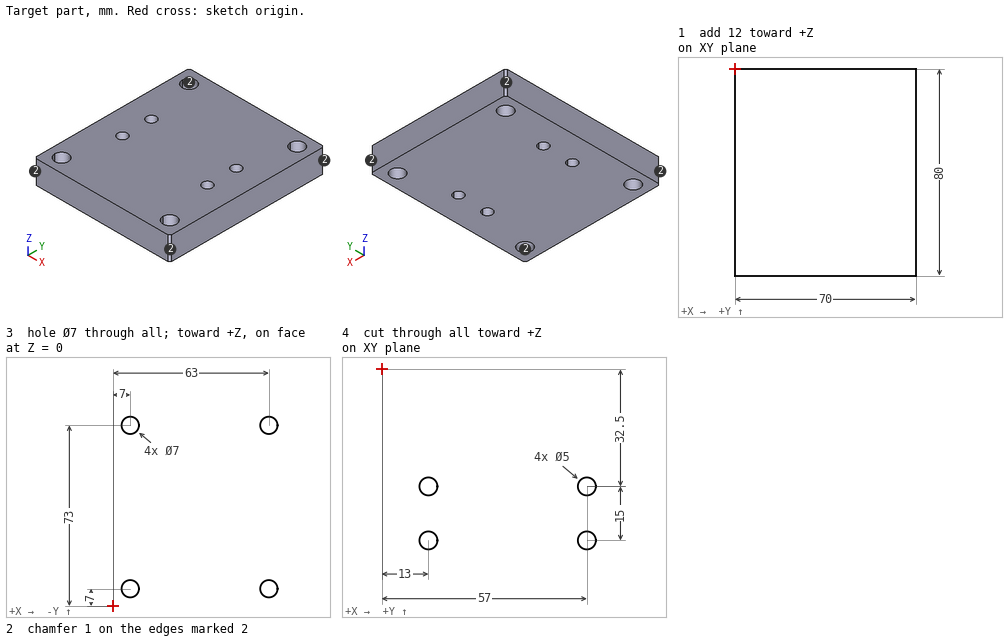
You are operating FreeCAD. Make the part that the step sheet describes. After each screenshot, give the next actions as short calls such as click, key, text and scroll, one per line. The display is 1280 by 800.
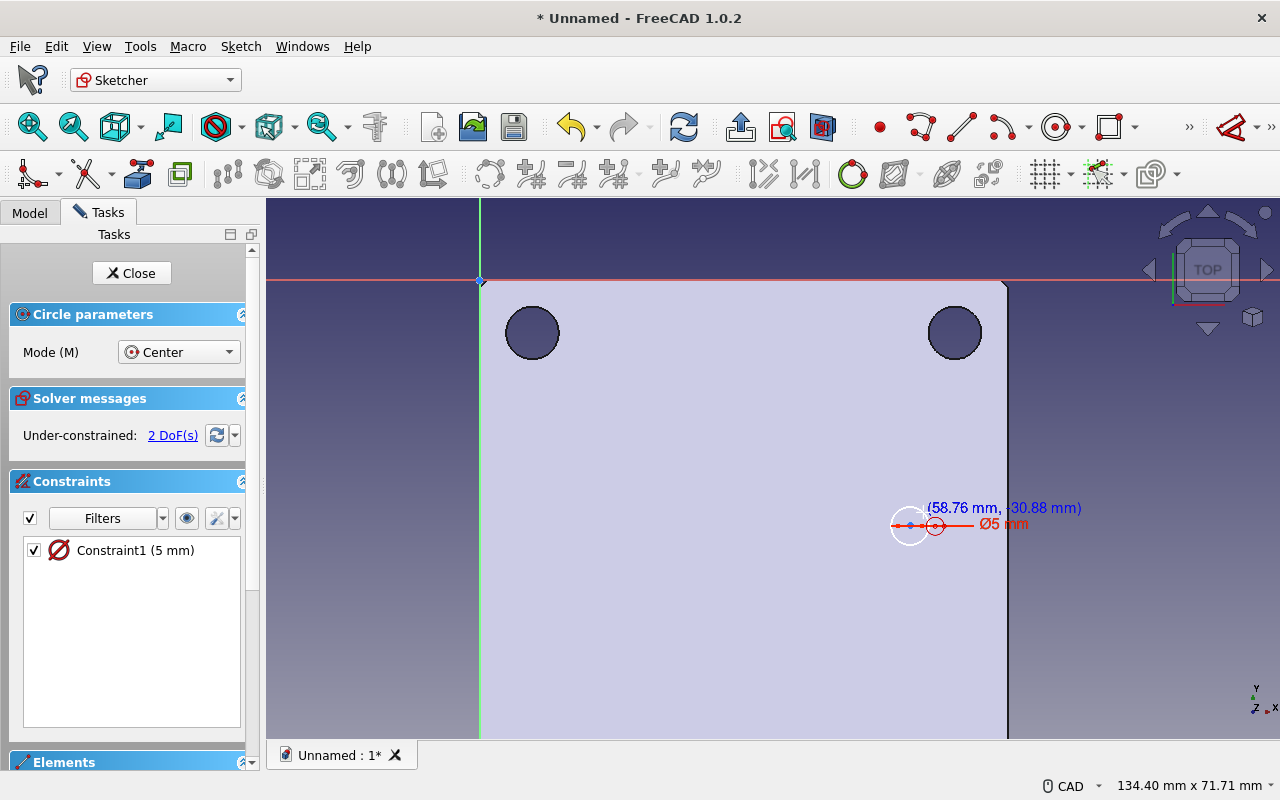
click(910, 638)
move(923, 625)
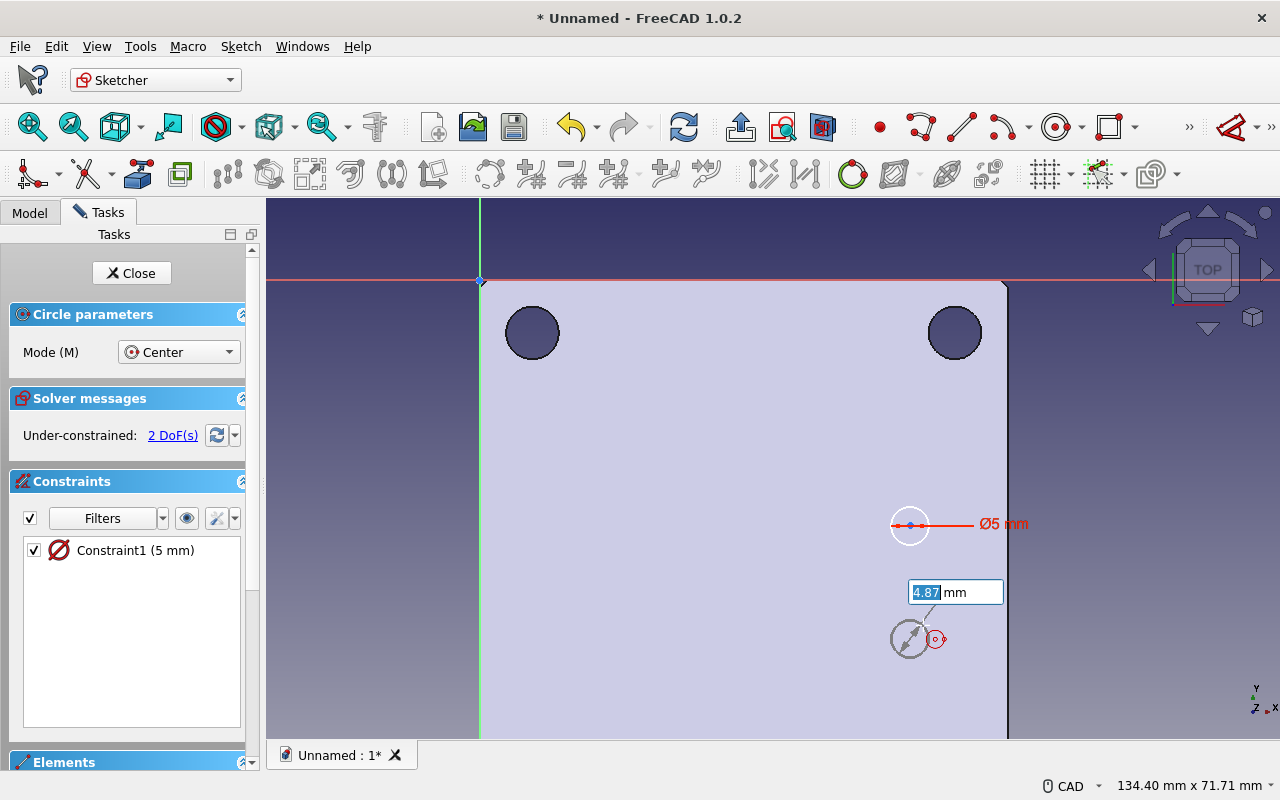
text(5)
key(Return)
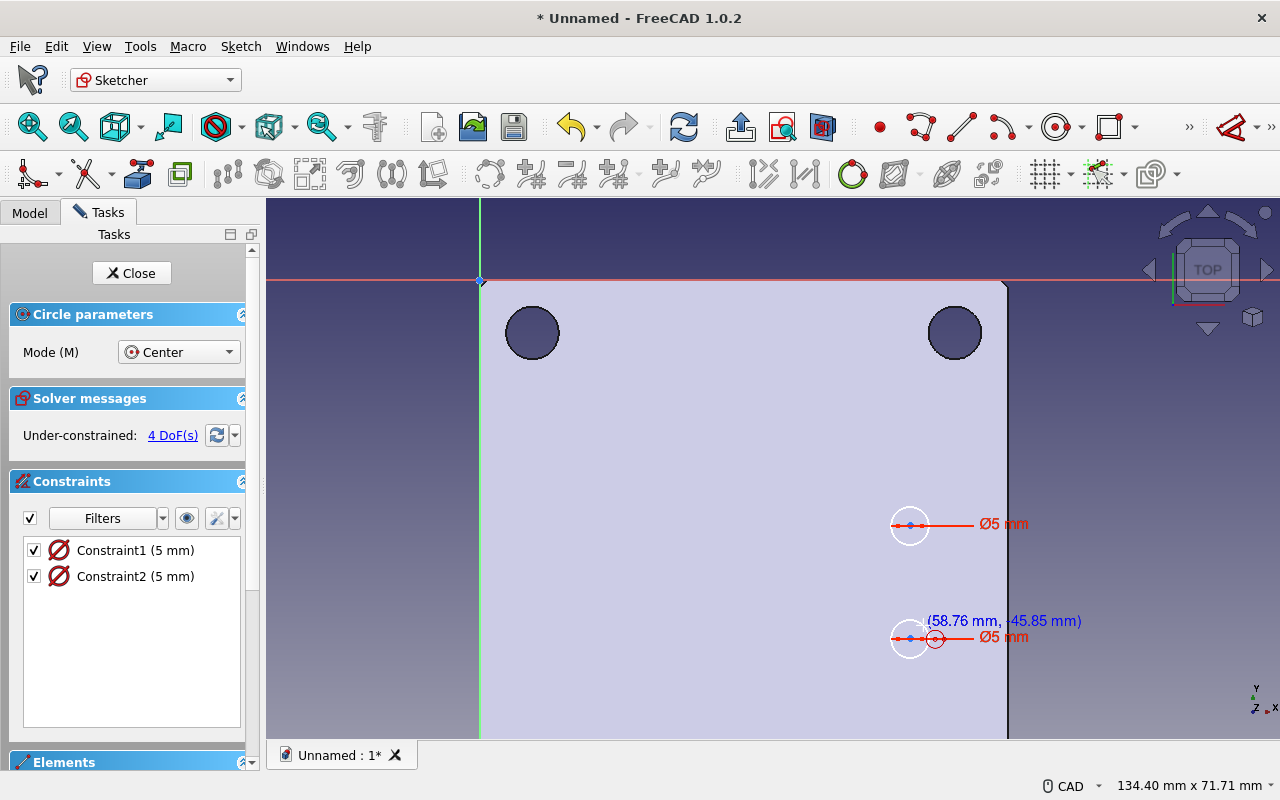
click(578, 638)
move(591, 625)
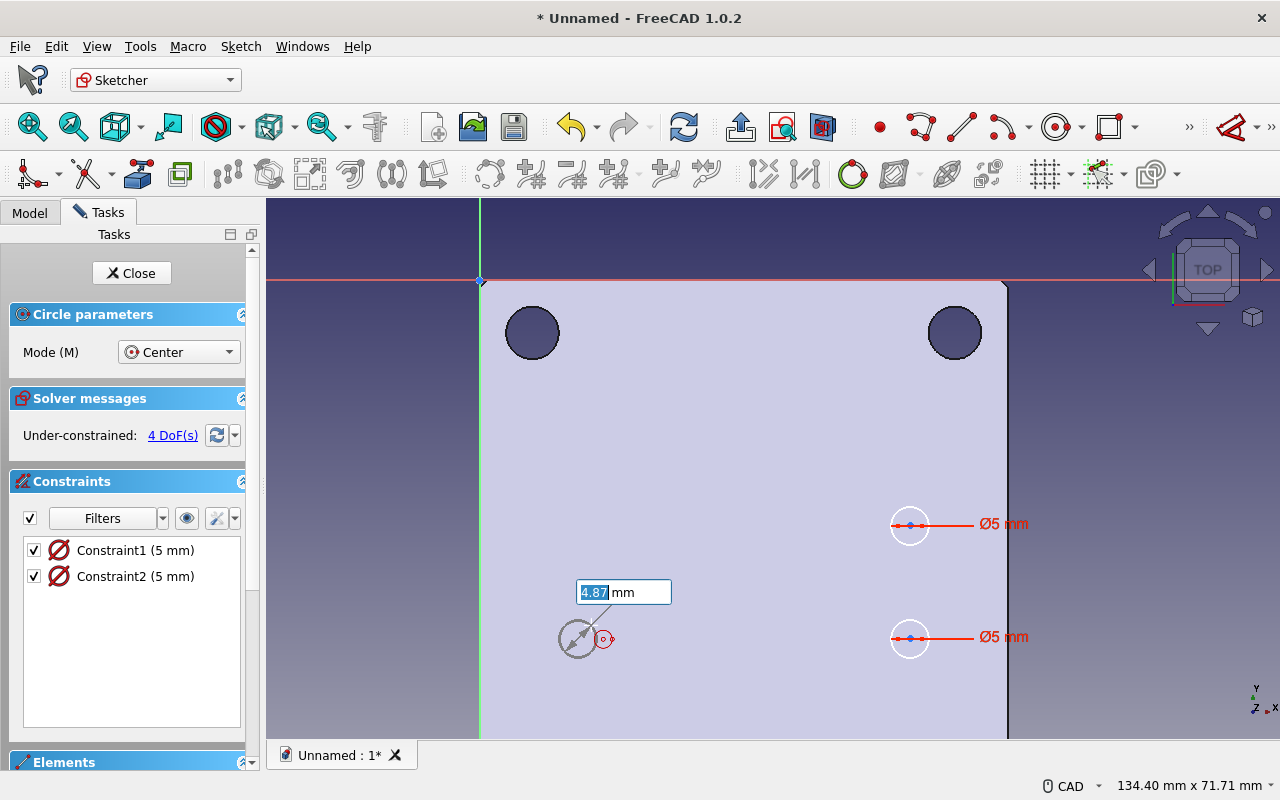
text(5)
key(Return)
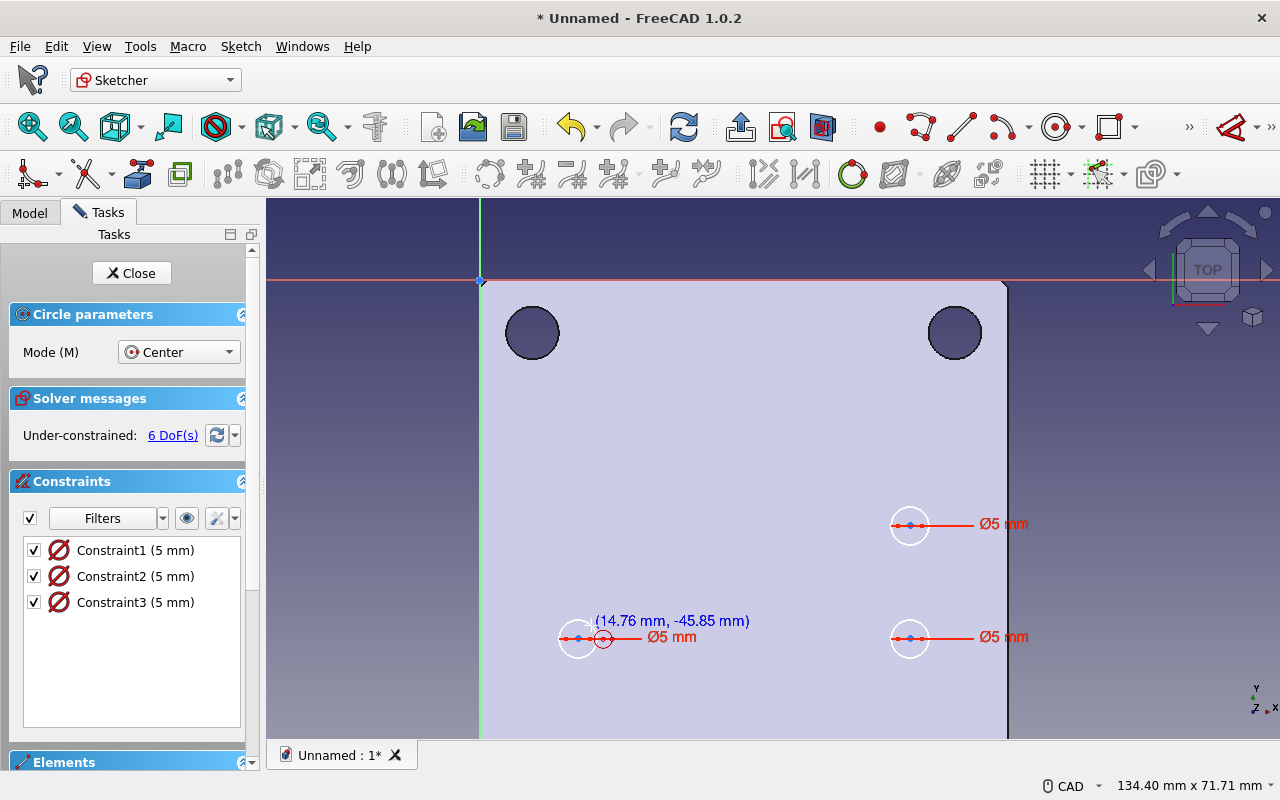
click(578, 525)
move(591, 512)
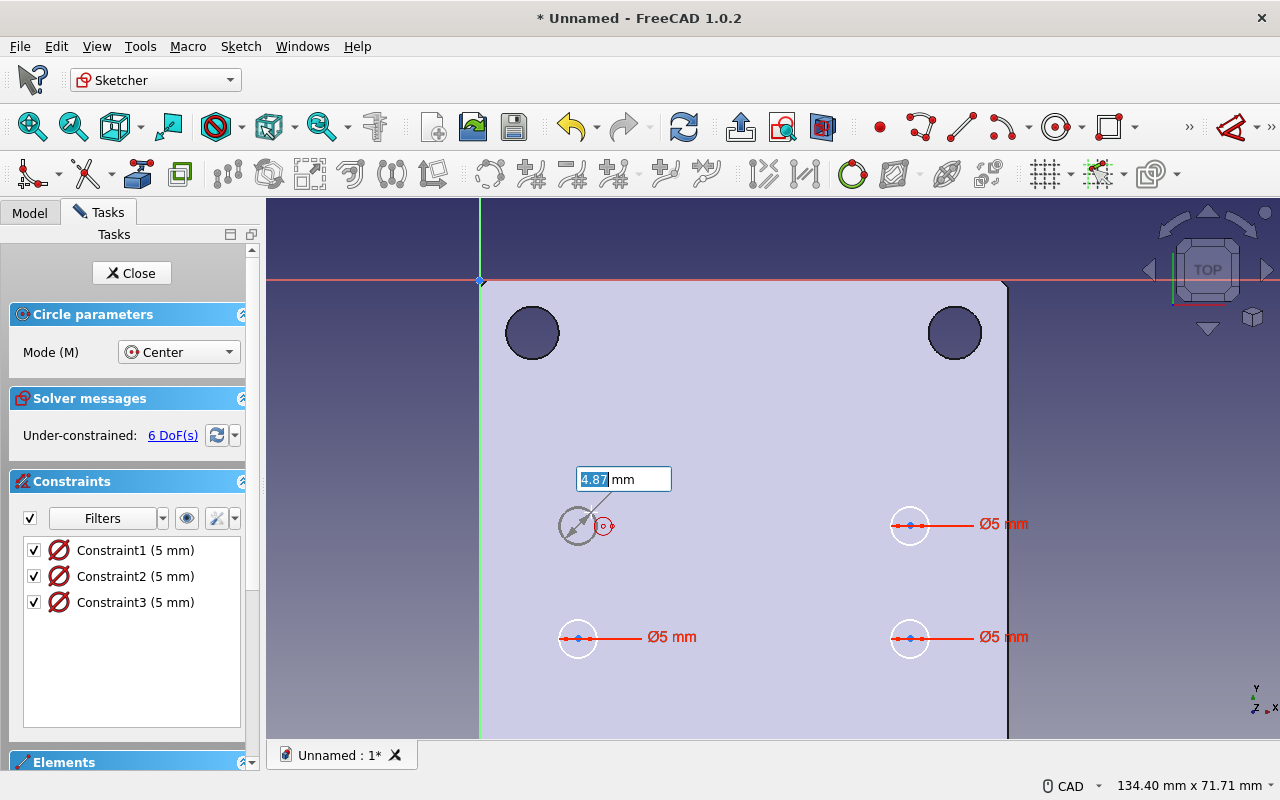
text(5)
key(Return)
key(Escape)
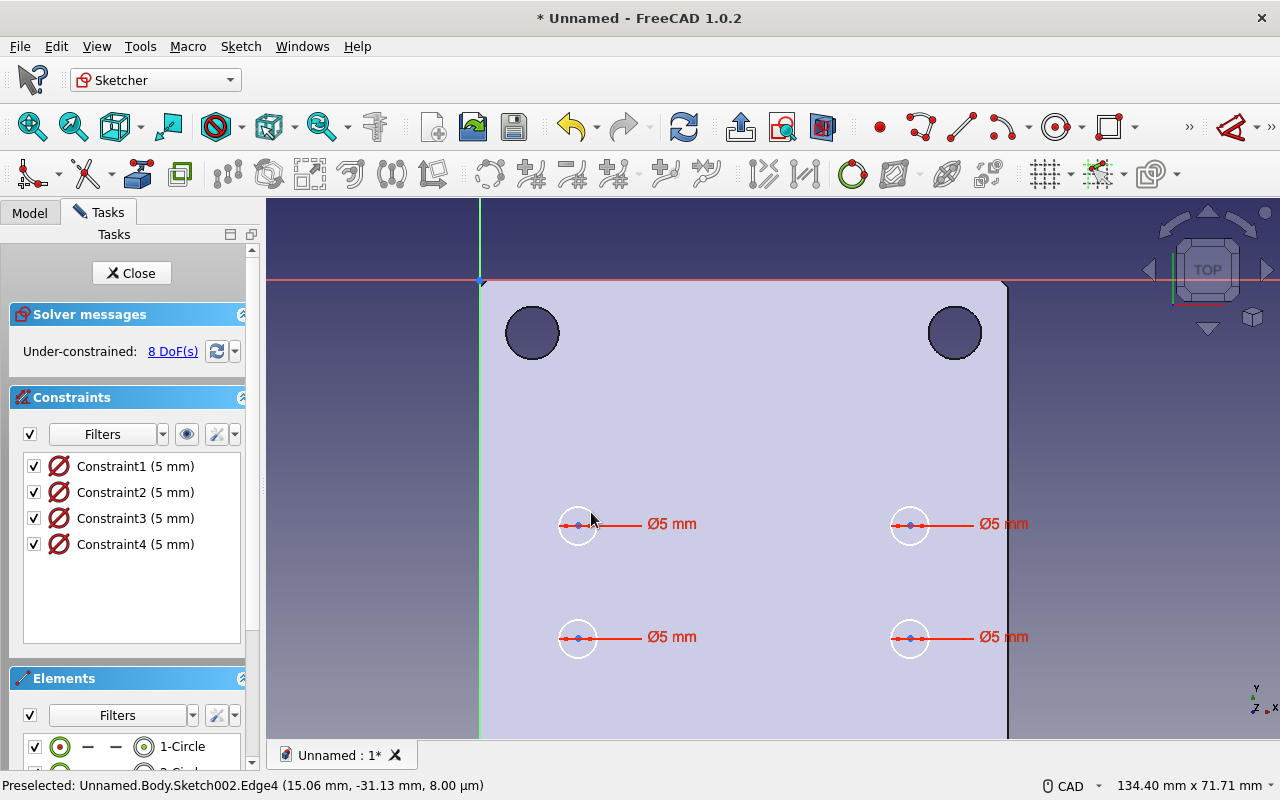
click(910, 526)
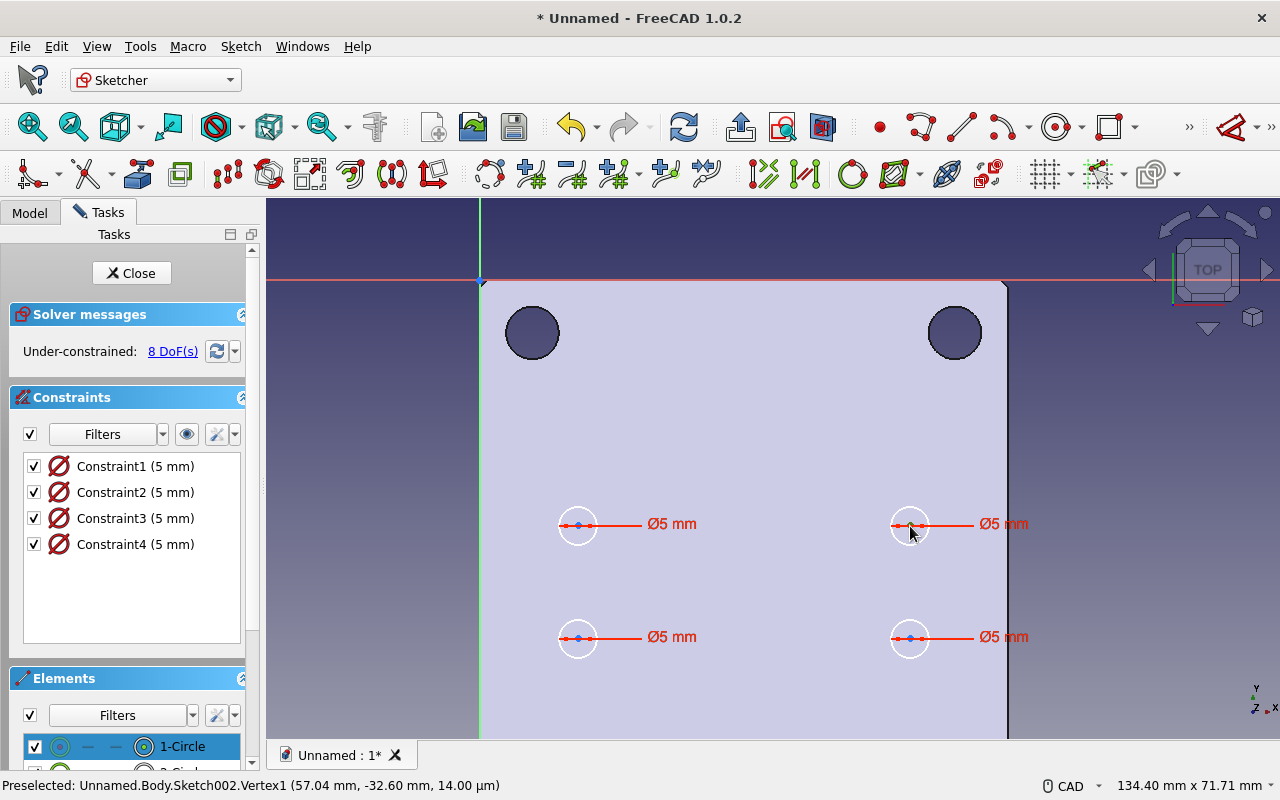
click(910, 639)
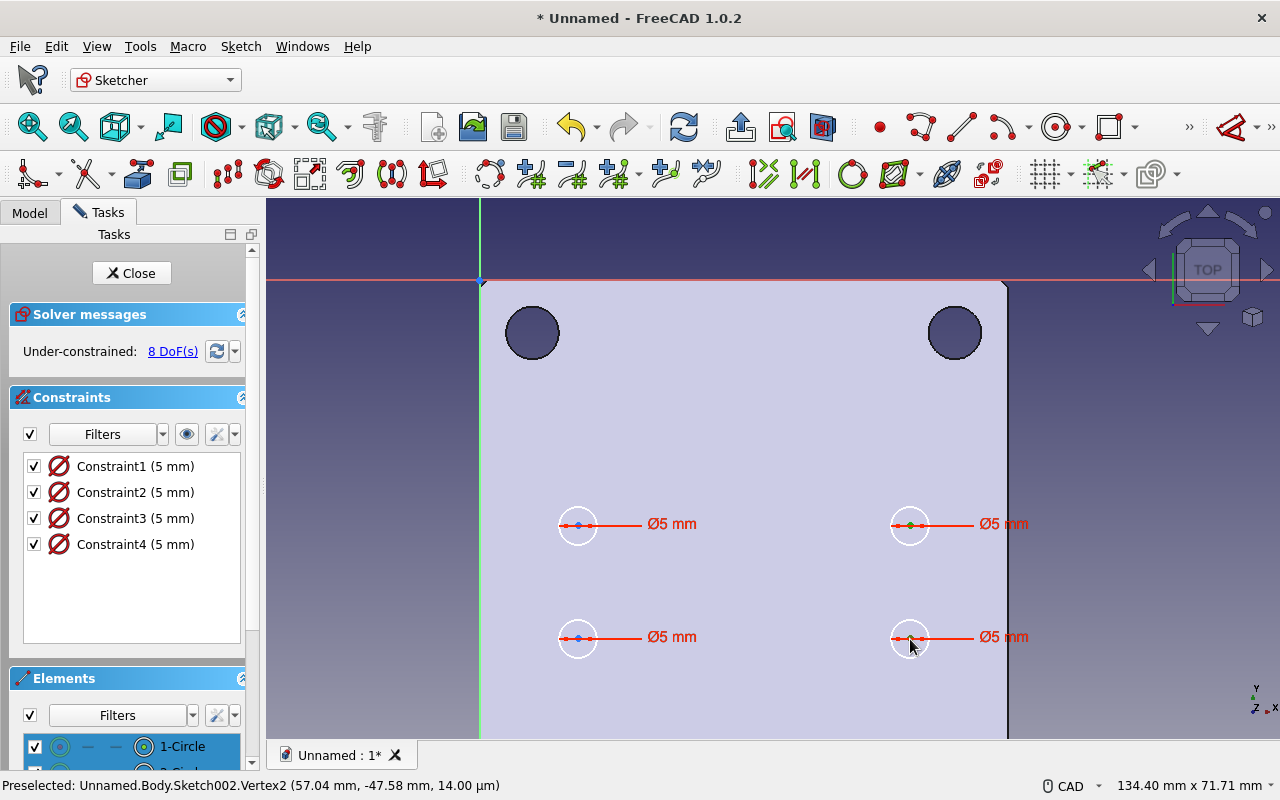
key(v)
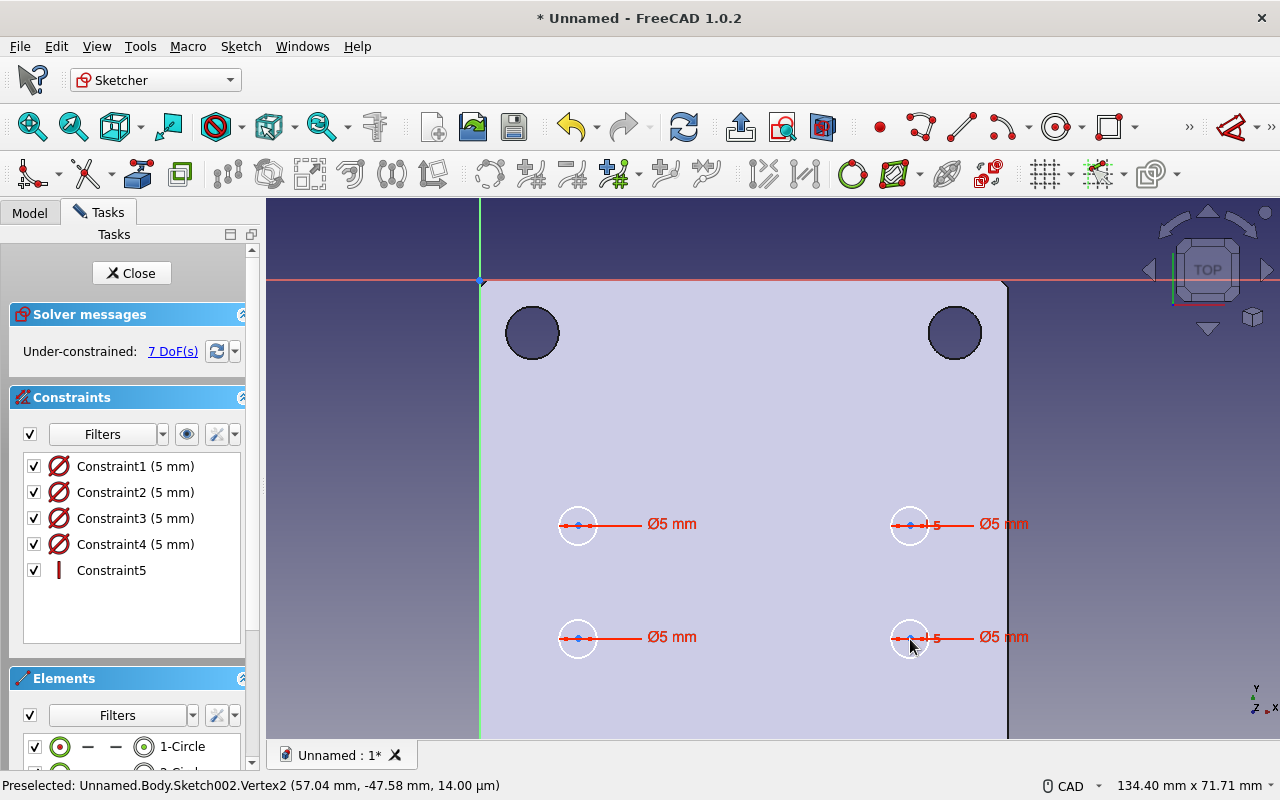
click(910, 639)